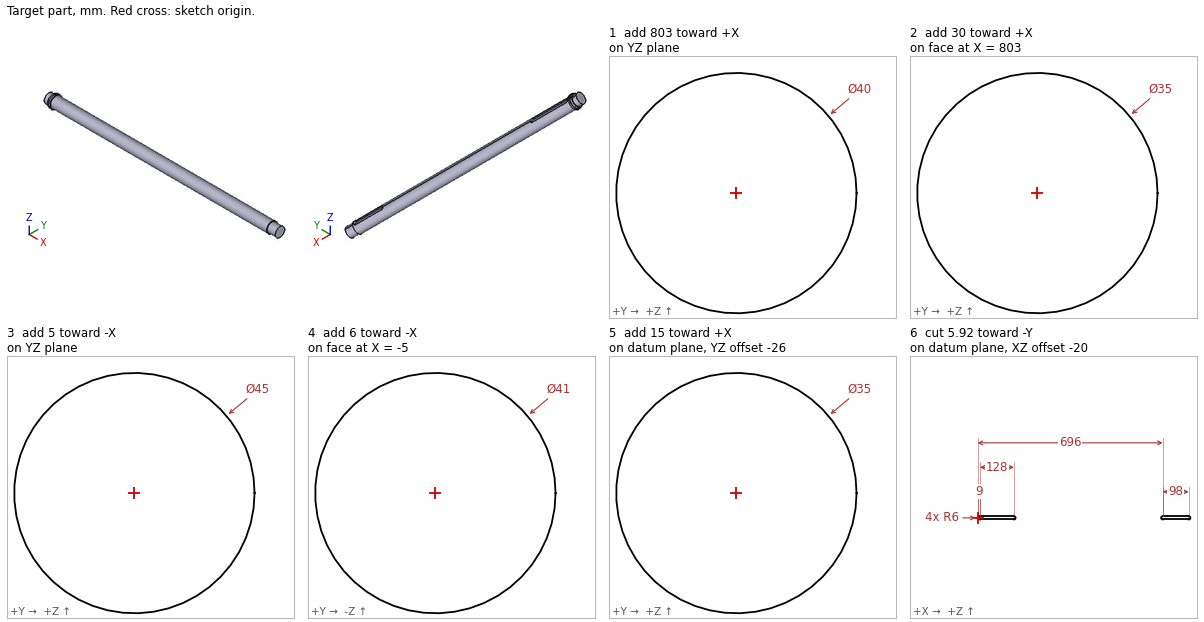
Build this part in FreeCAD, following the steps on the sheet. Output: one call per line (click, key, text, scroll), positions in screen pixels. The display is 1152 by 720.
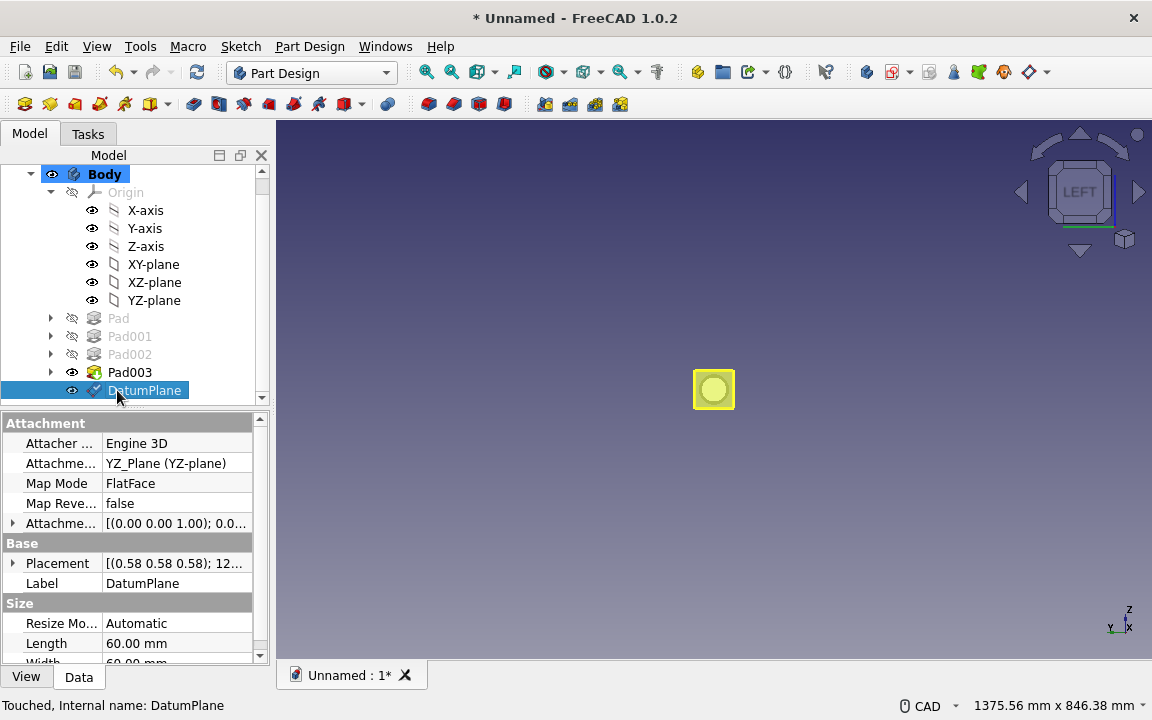
click(892, 72)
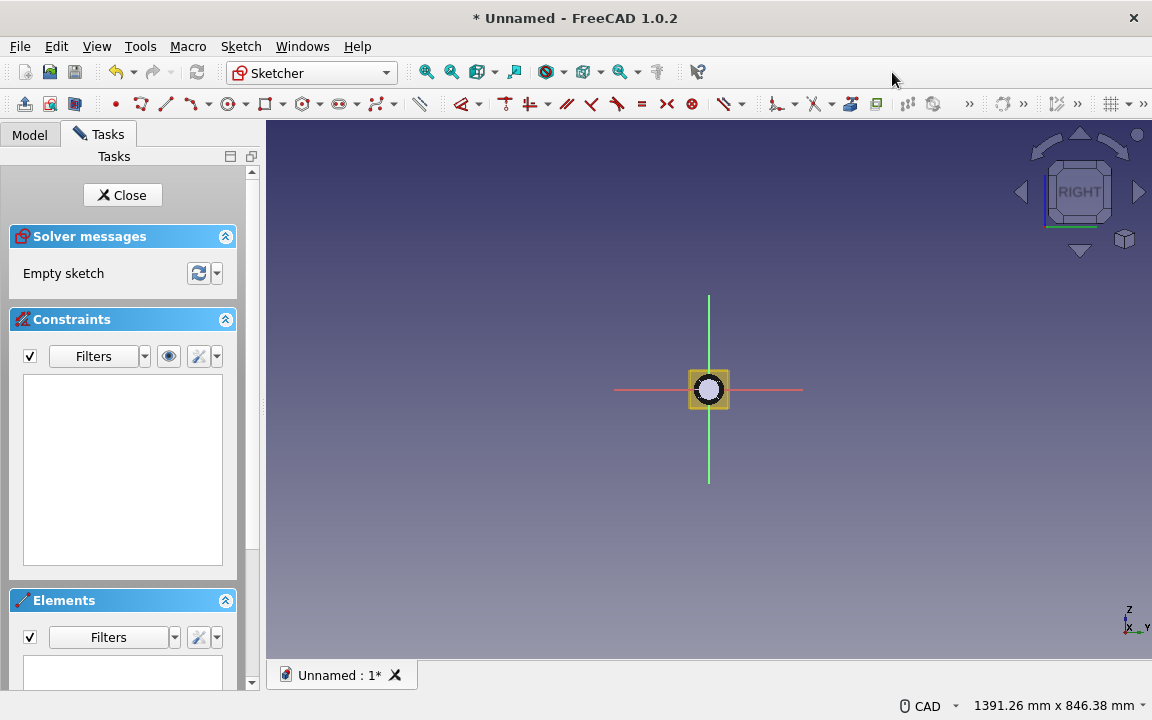
click(75, 104)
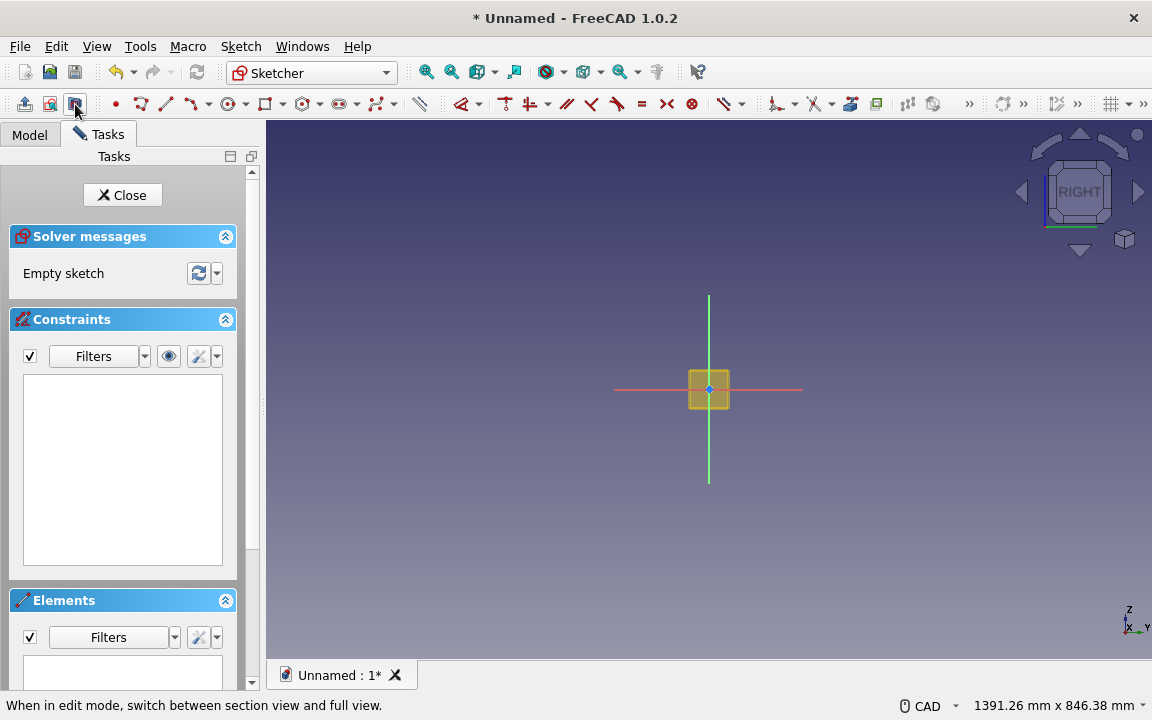
scroll(713, 390, up, 14)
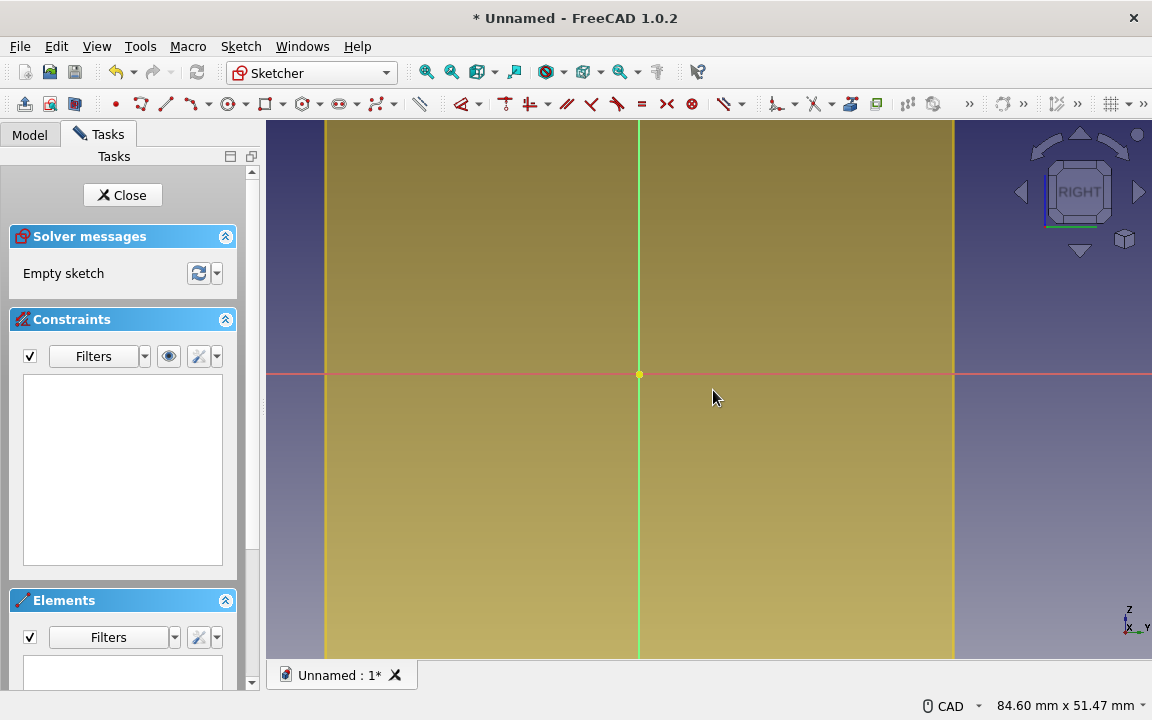
click(228, 104)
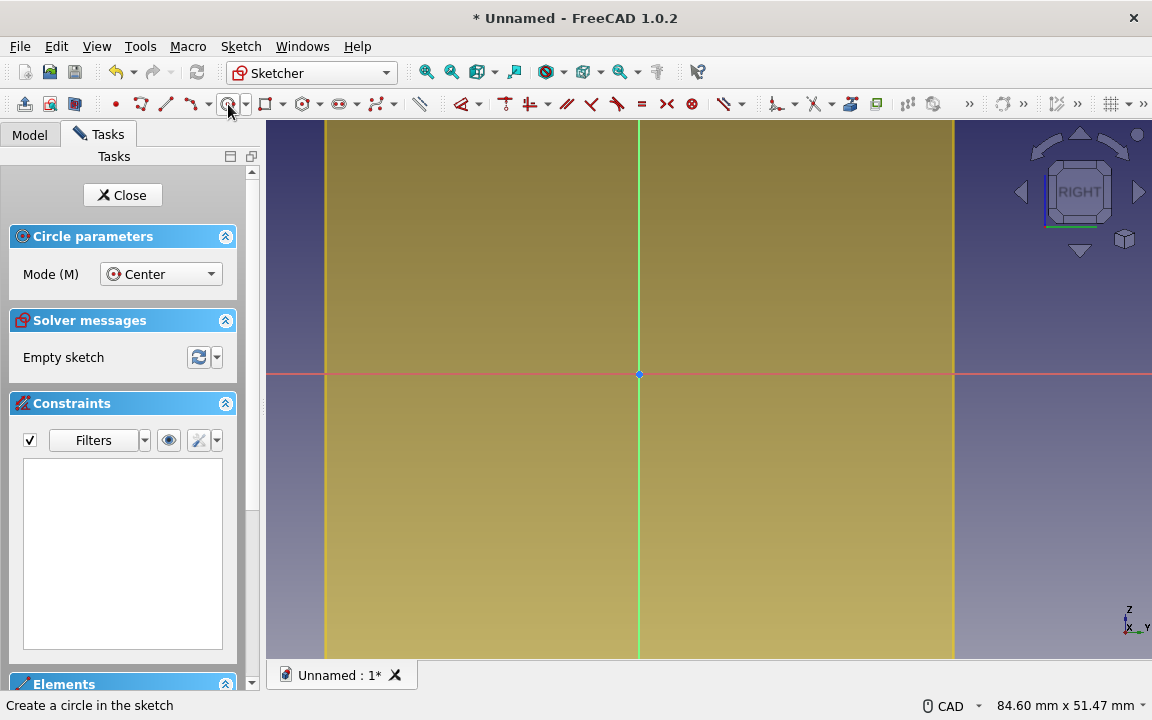
click(639, 374)
move(769, 244)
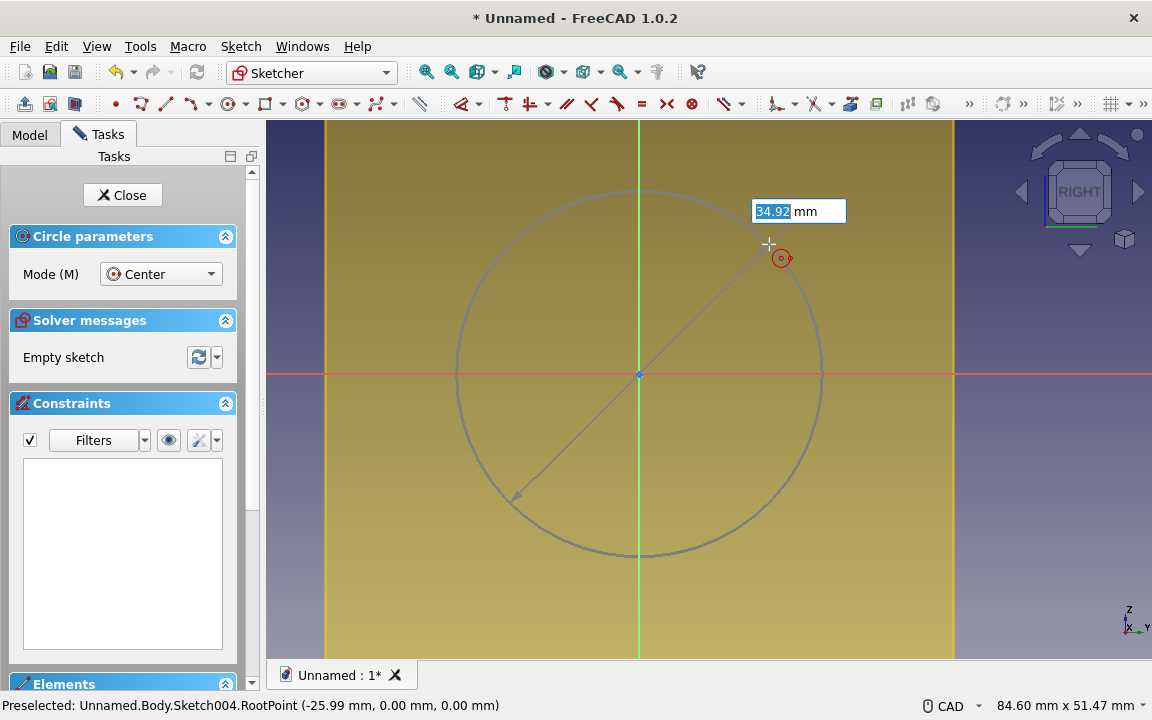
text(35)
key(Return)
key(Escape)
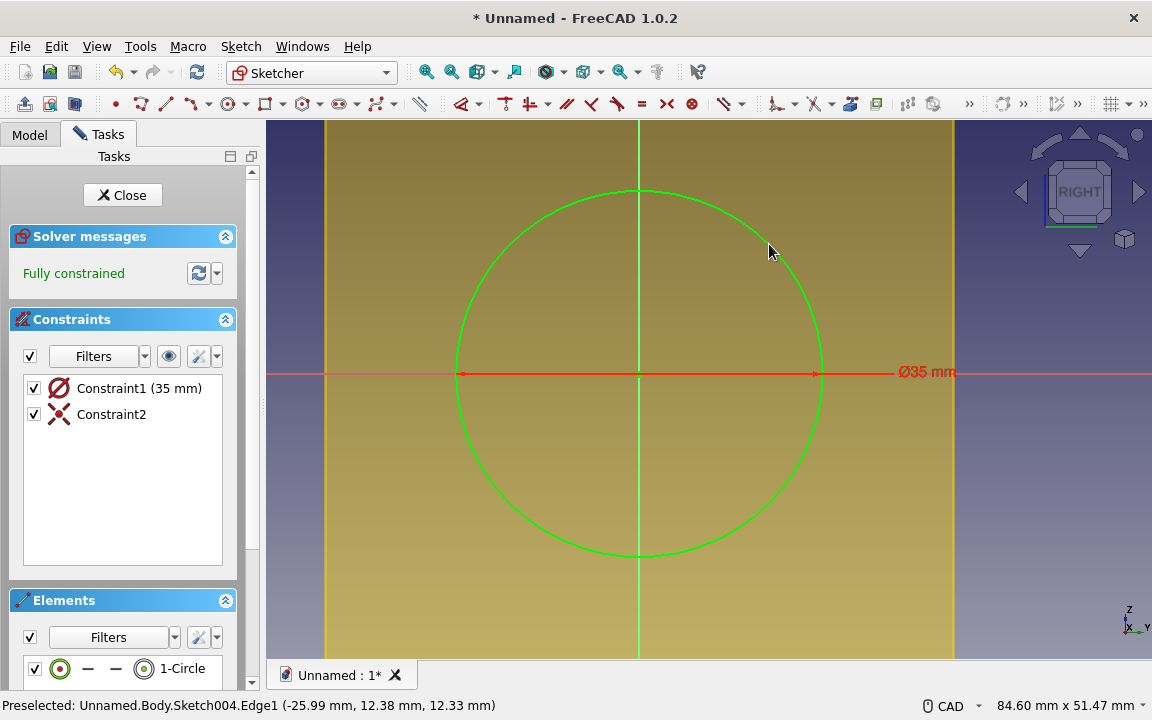
click(123, 195)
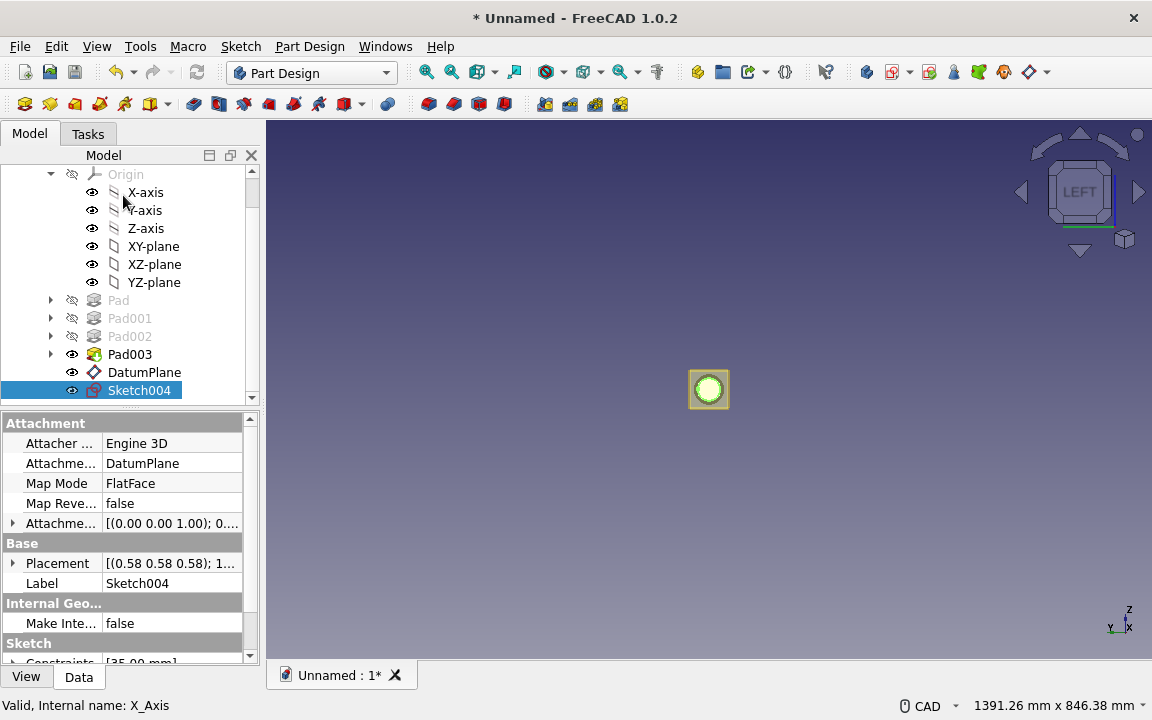
click(25, 104)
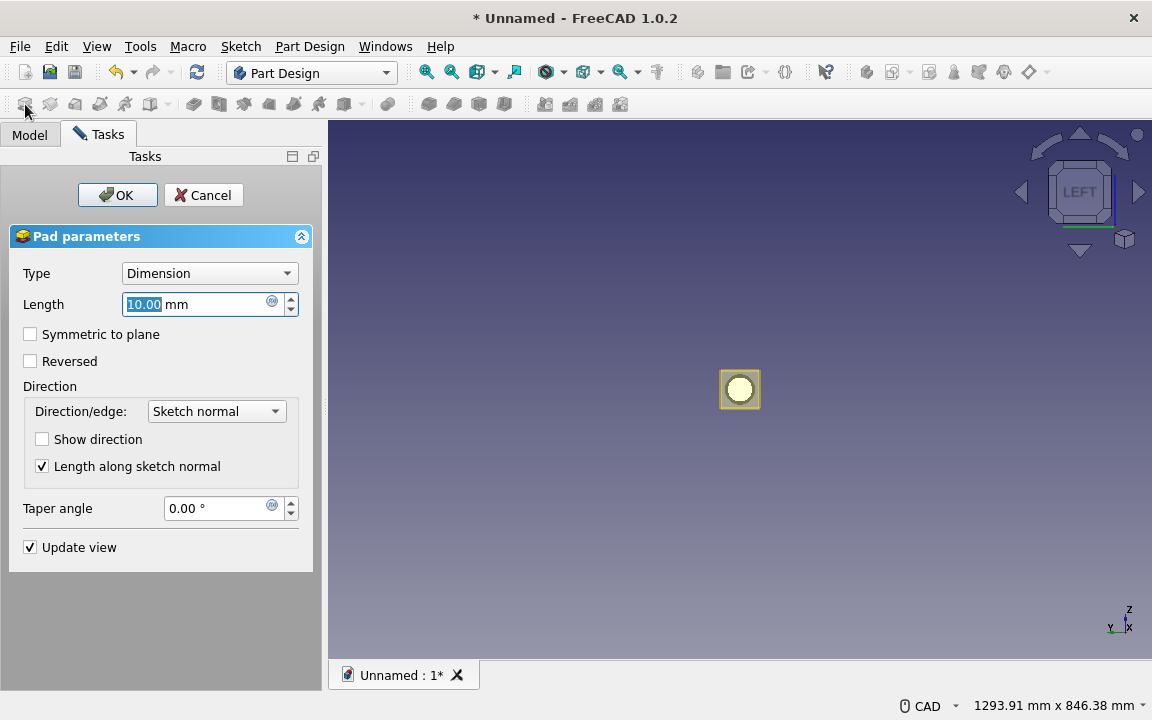
text(15)
key(Tab)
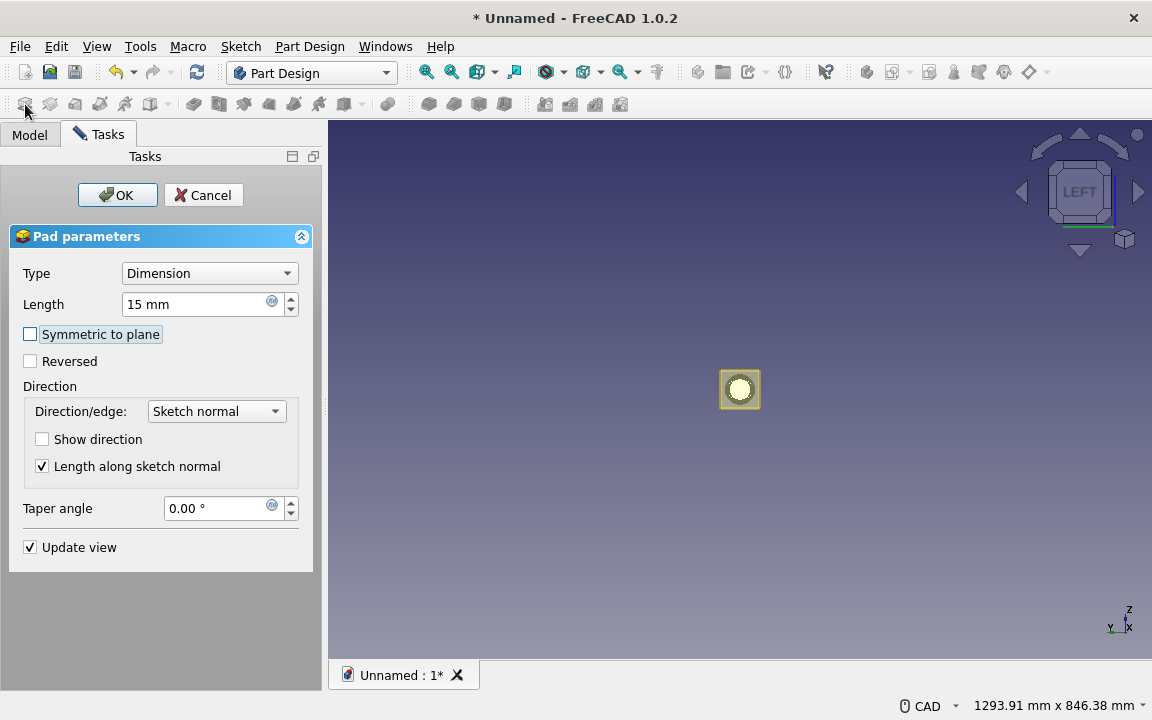
click(118, 195)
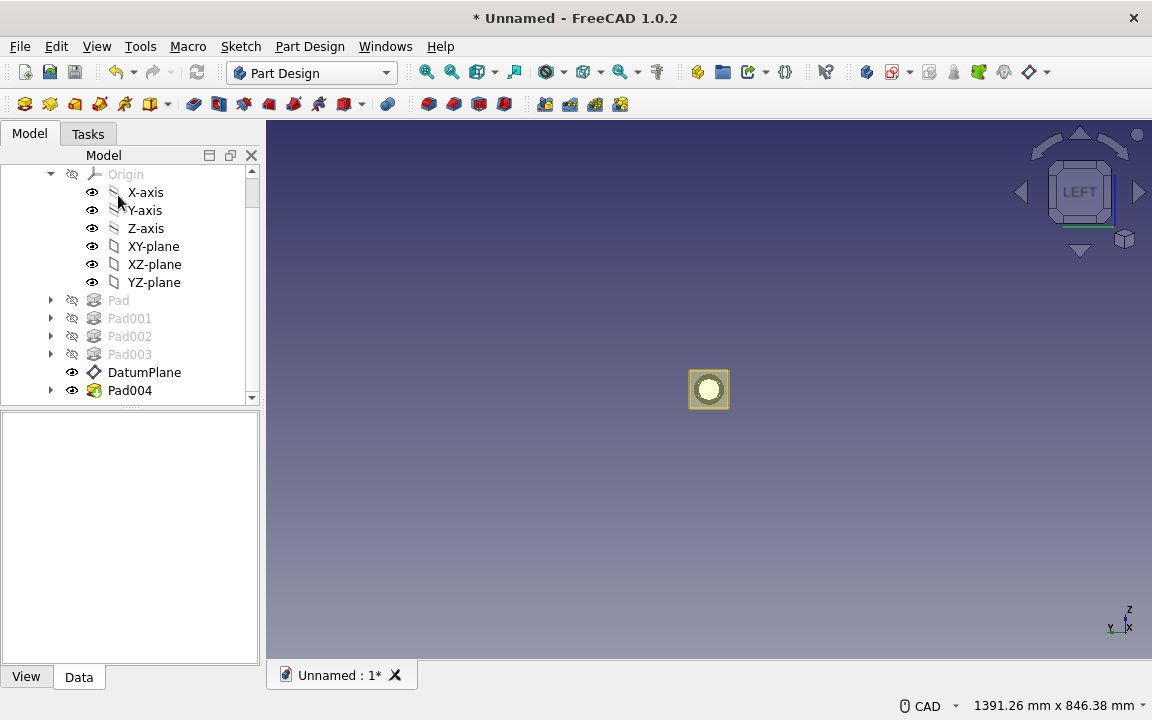
click(117, 372)
key(space)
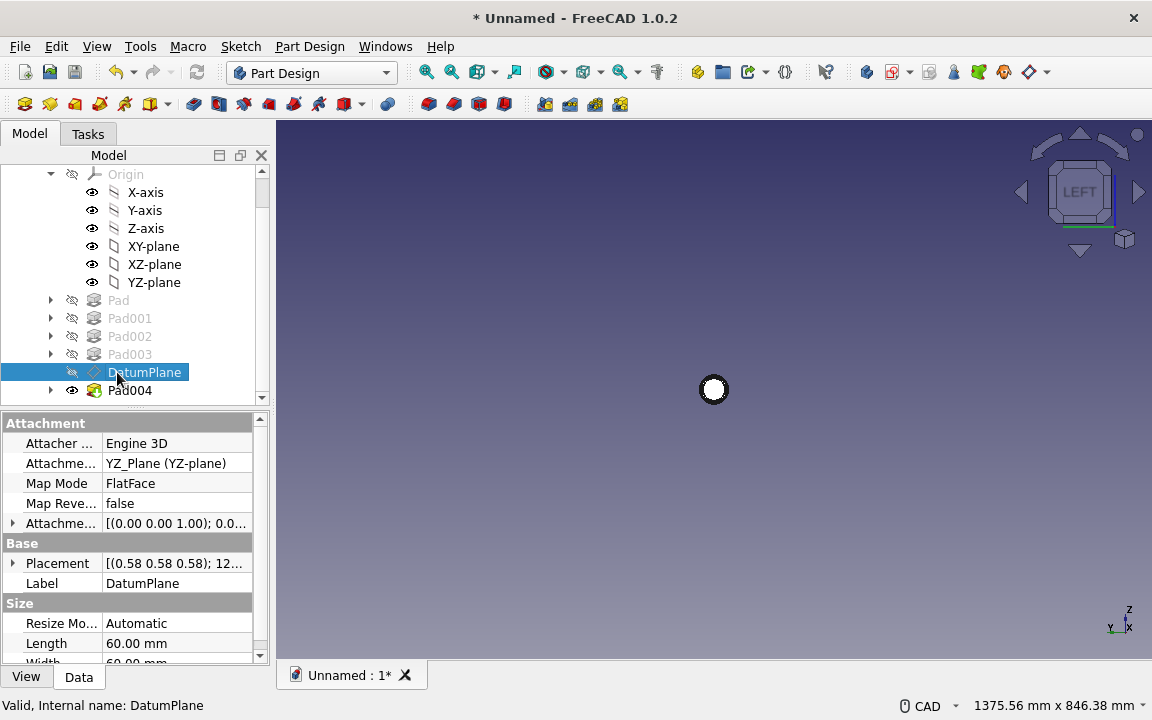
key(v)
key(f)